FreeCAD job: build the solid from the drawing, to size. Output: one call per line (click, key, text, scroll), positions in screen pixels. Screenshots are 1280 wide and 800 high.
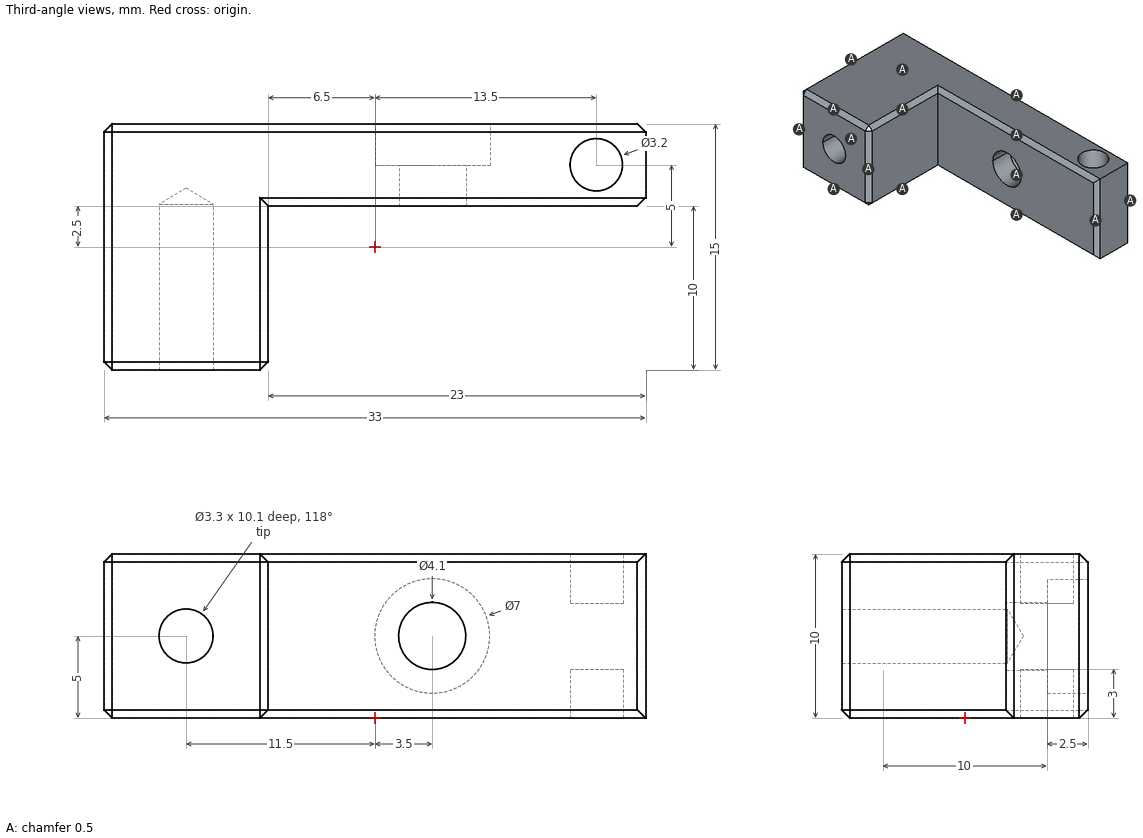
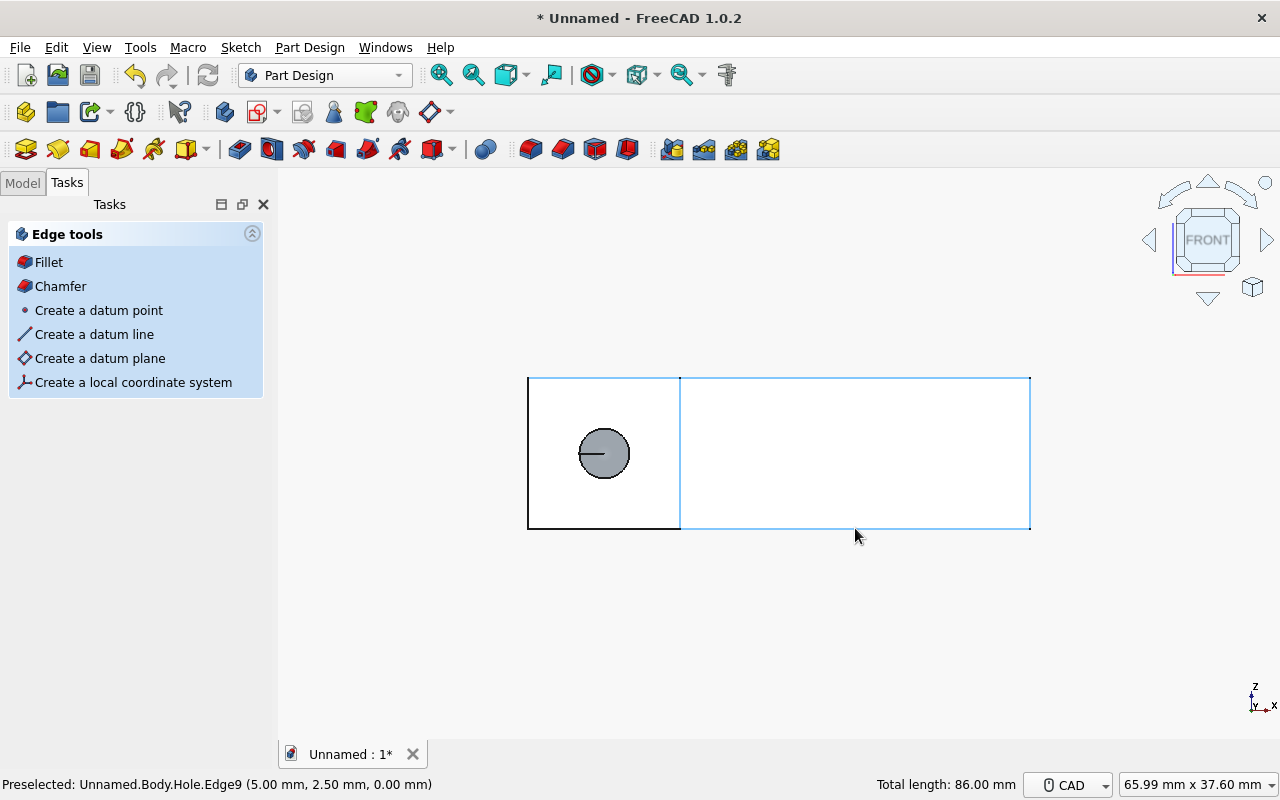
click(604, 528, ctrl)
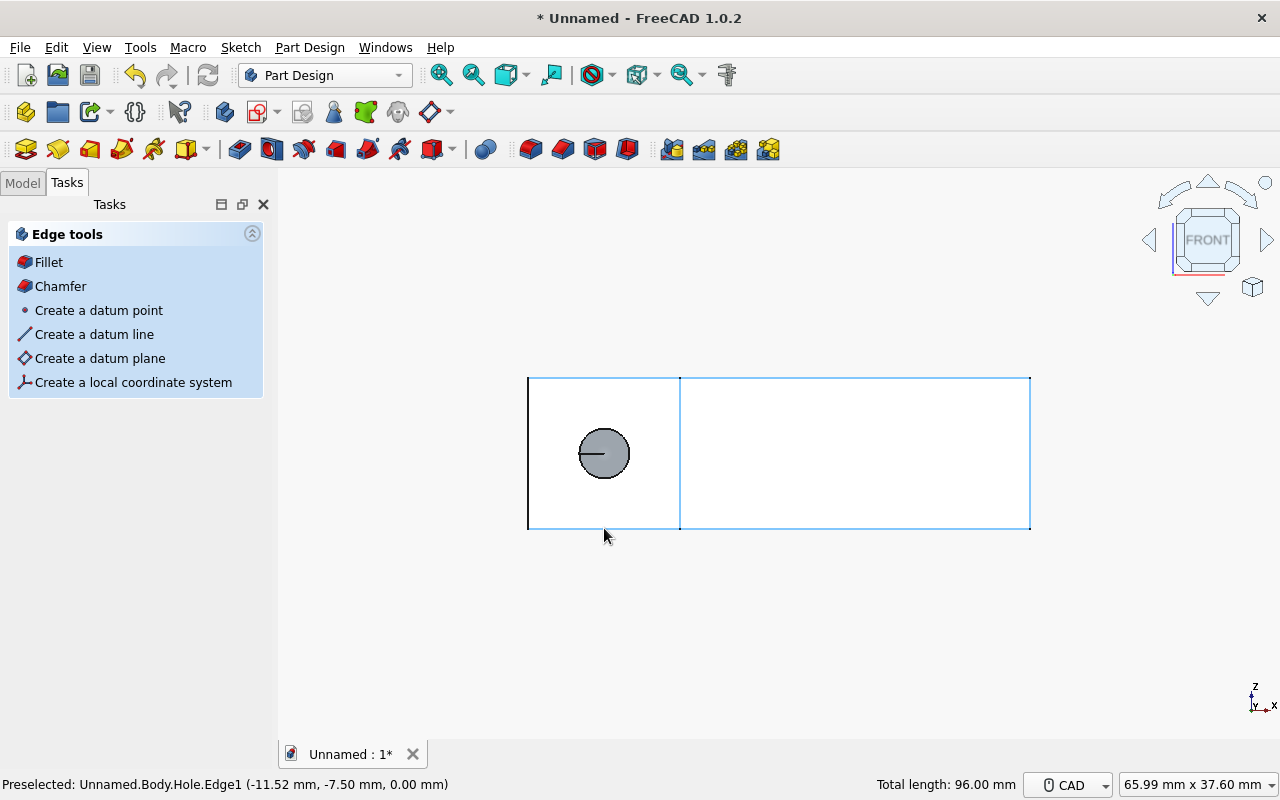
key(3)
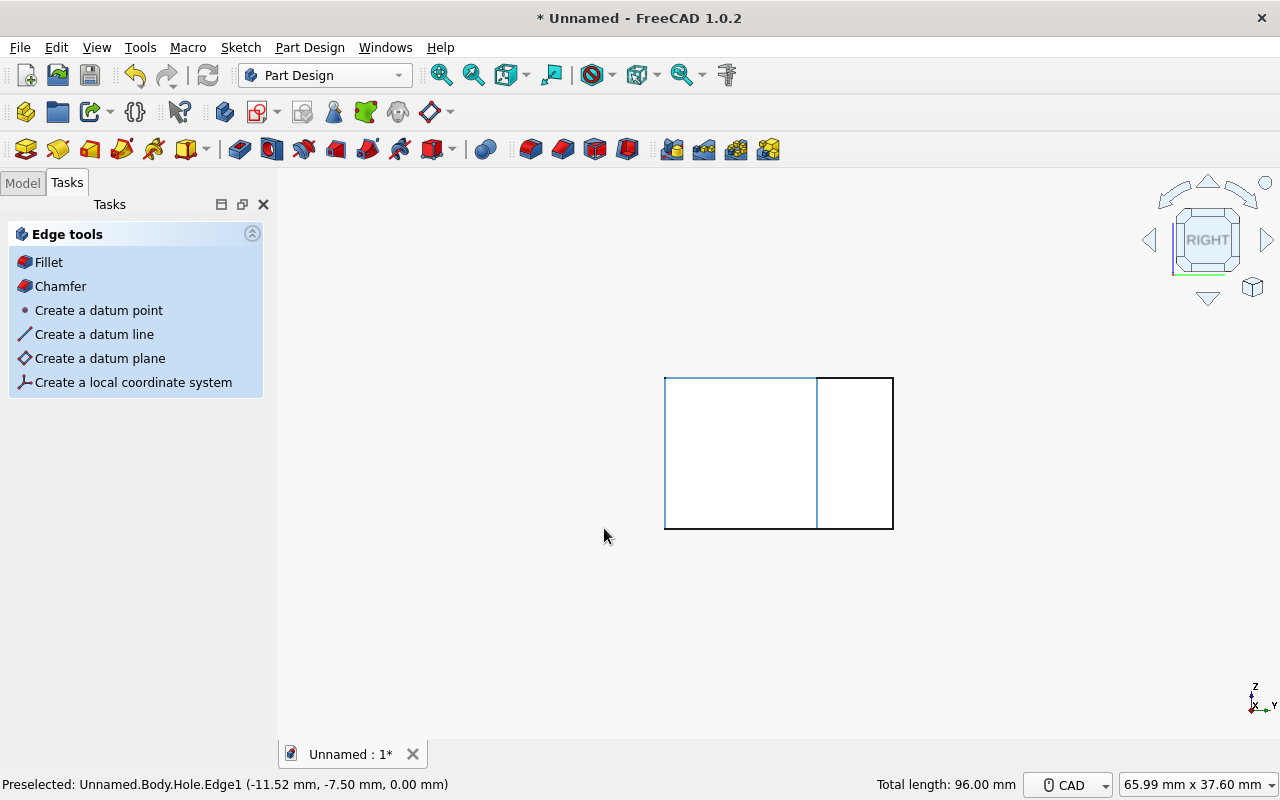
click(442, 76)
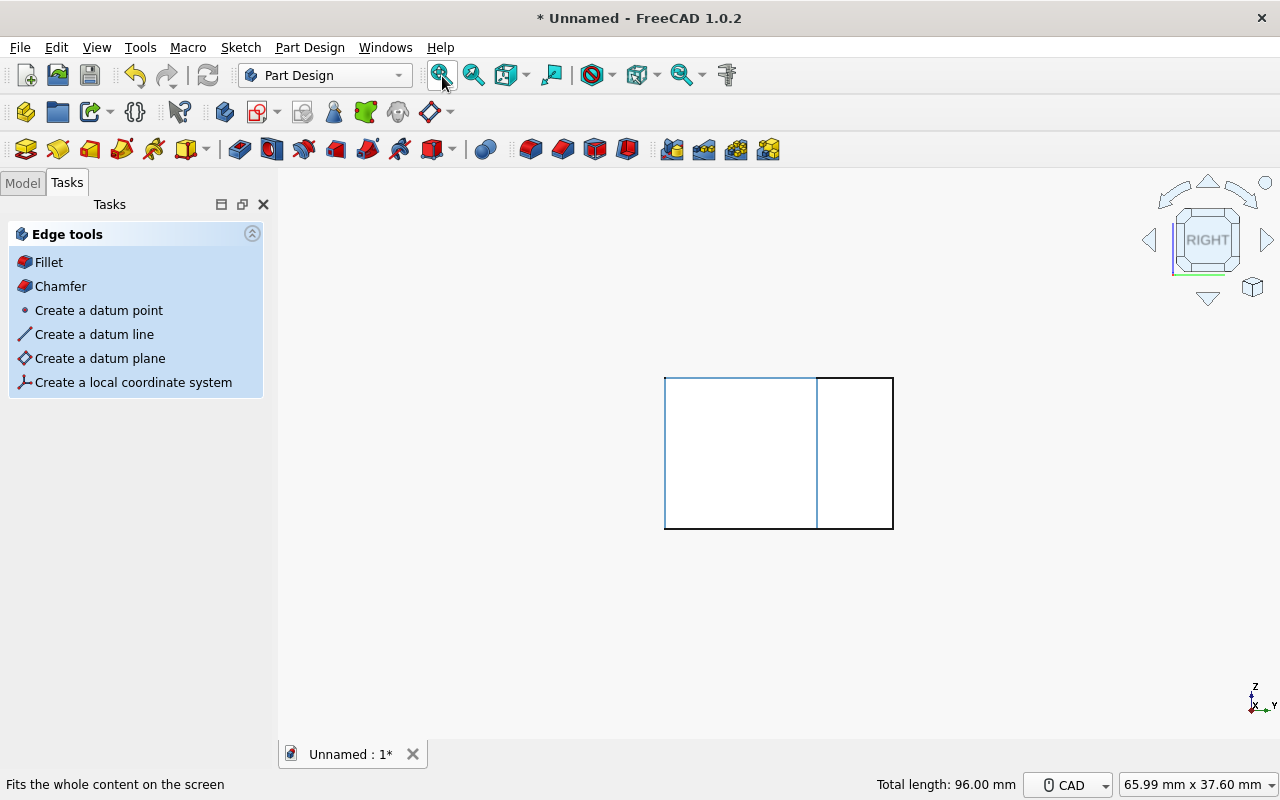
click(741, 528, ctrl)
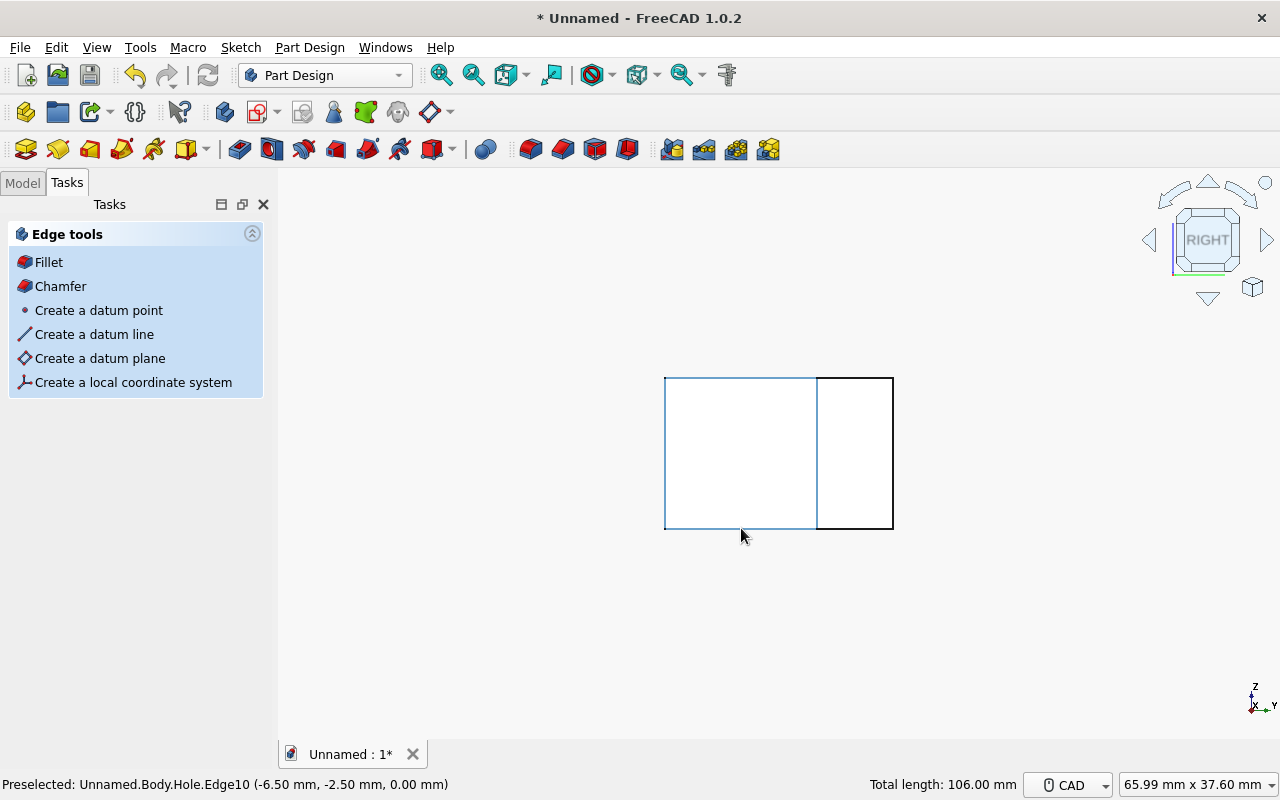
key(5)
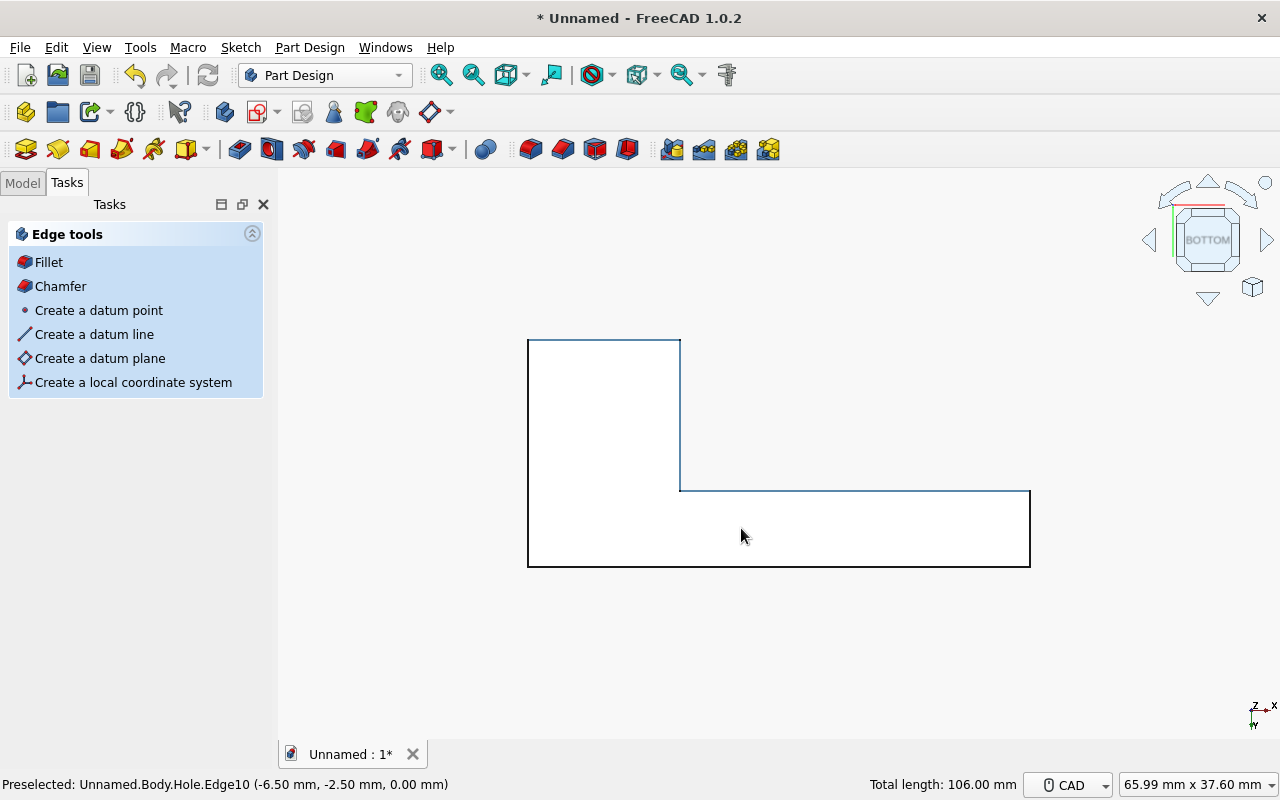
key(4)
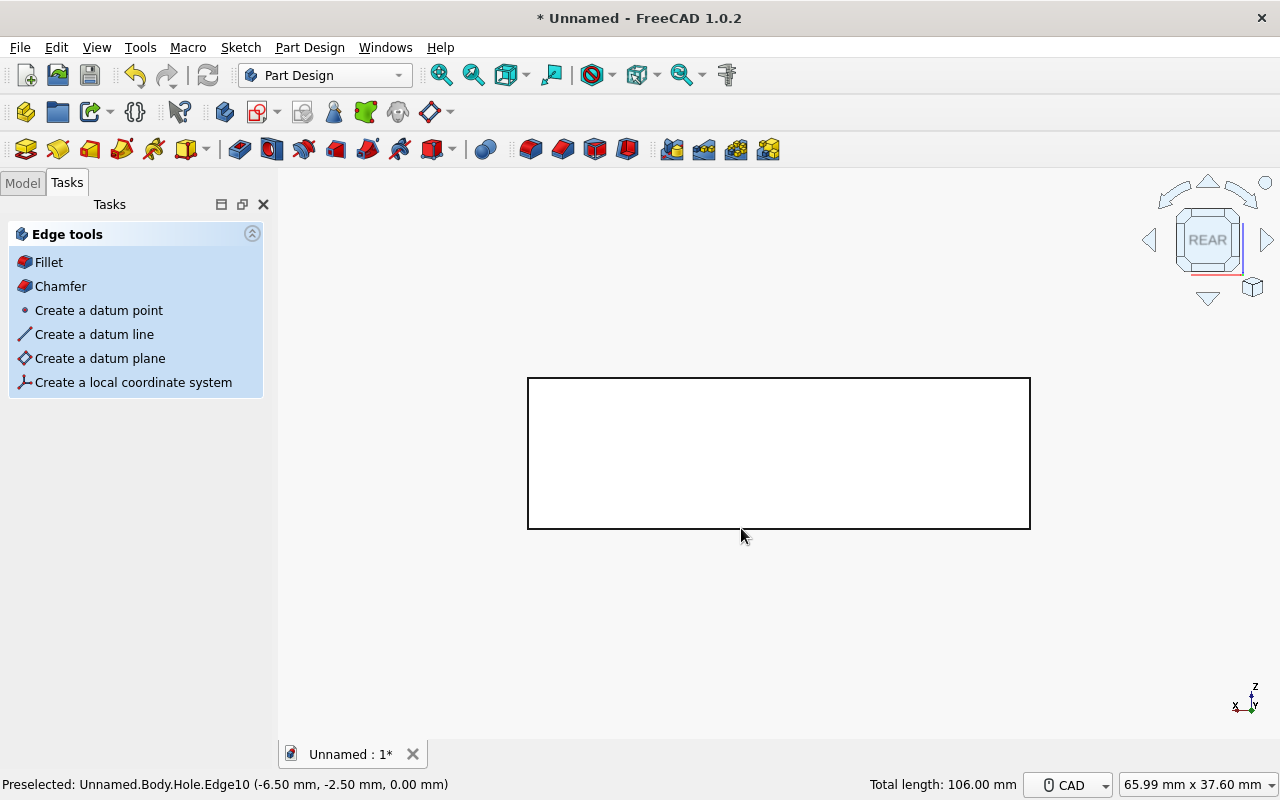
click(636, 452, ctrl)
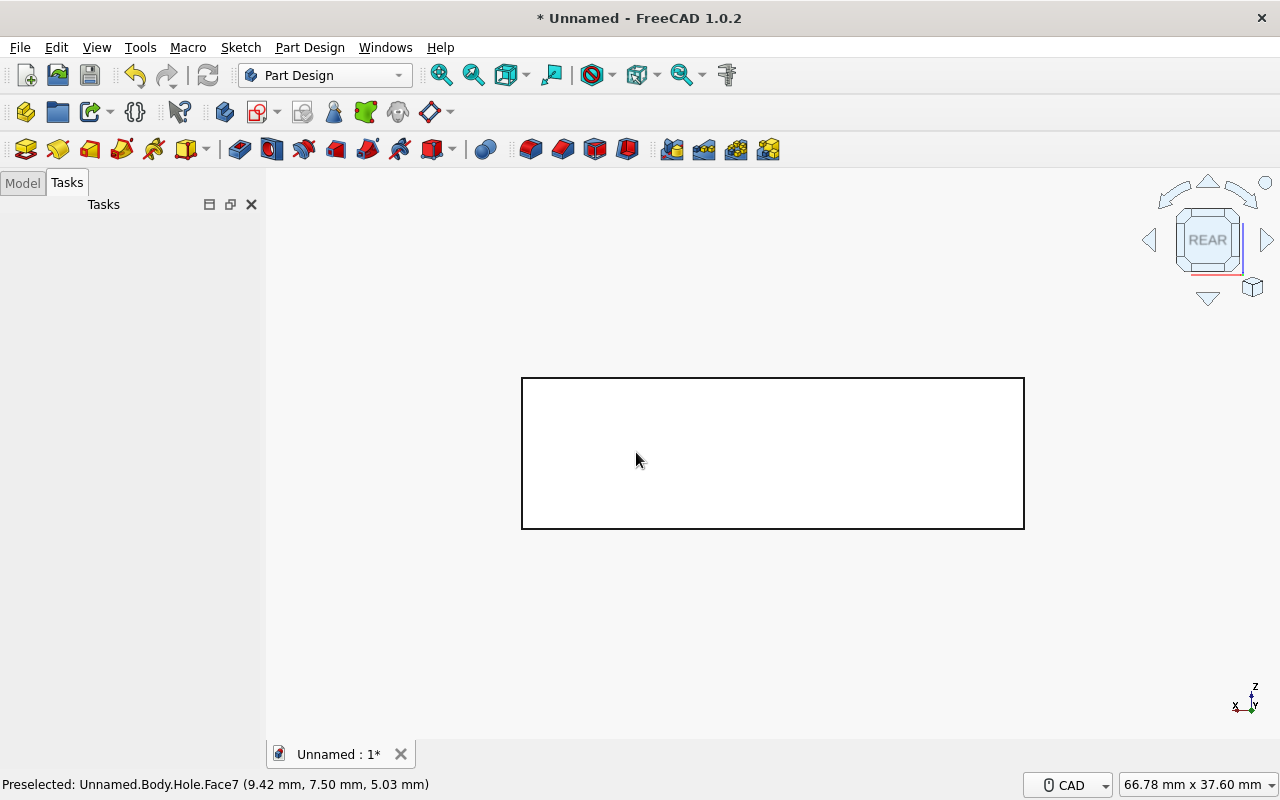
key(6)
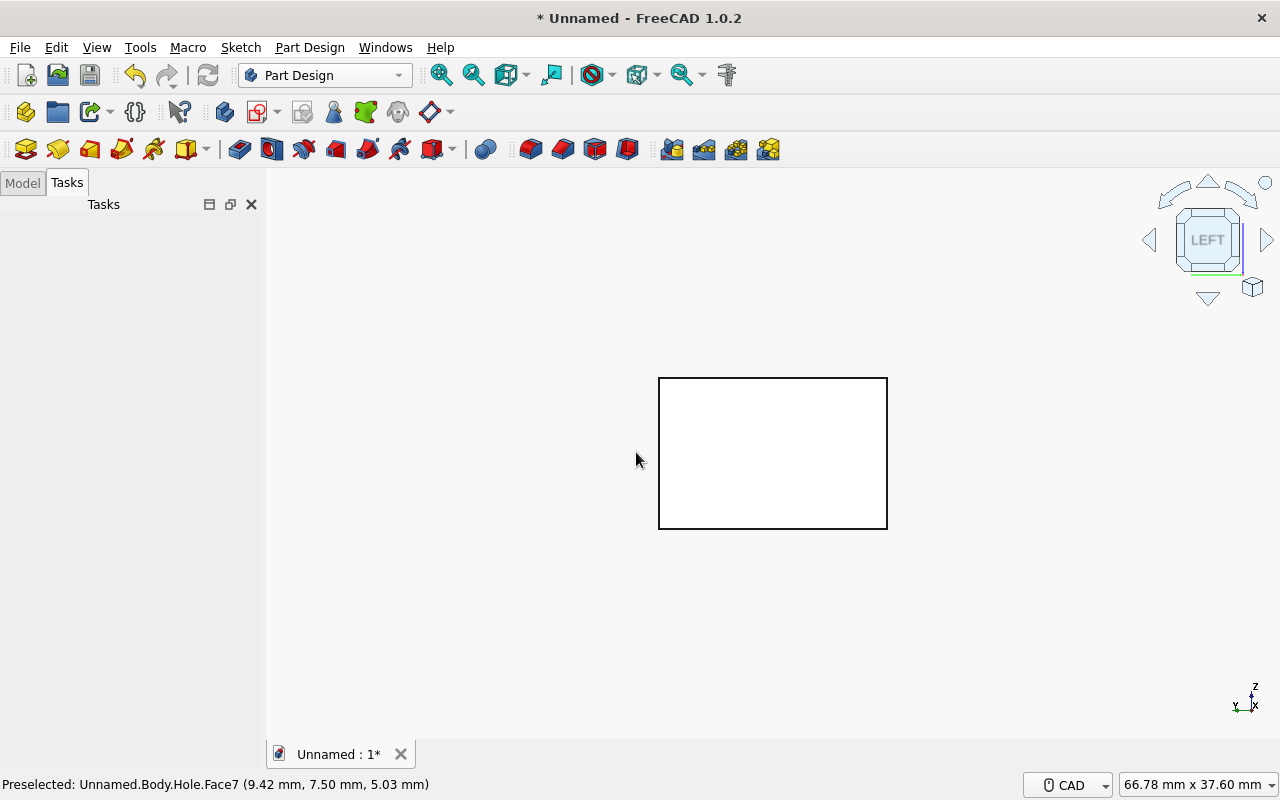
click(442, 76)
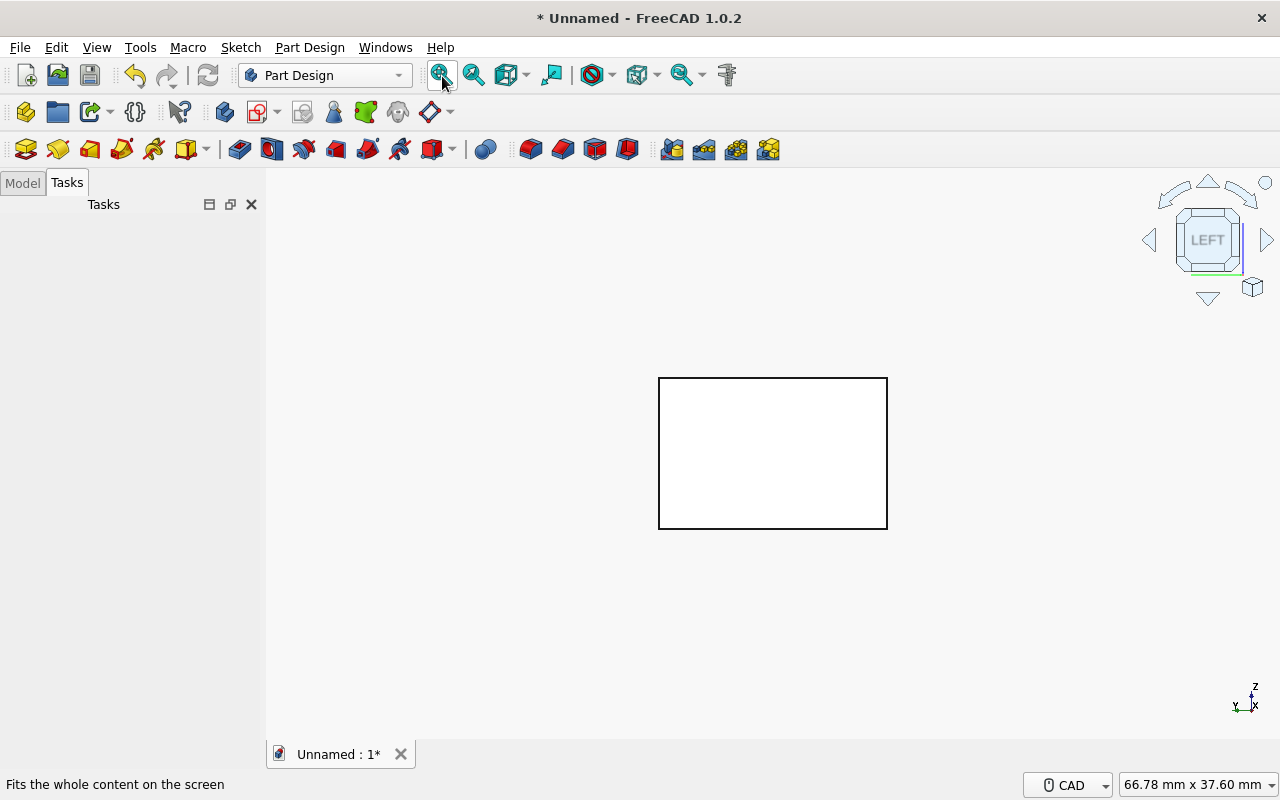
click(740, 452, ctrl)